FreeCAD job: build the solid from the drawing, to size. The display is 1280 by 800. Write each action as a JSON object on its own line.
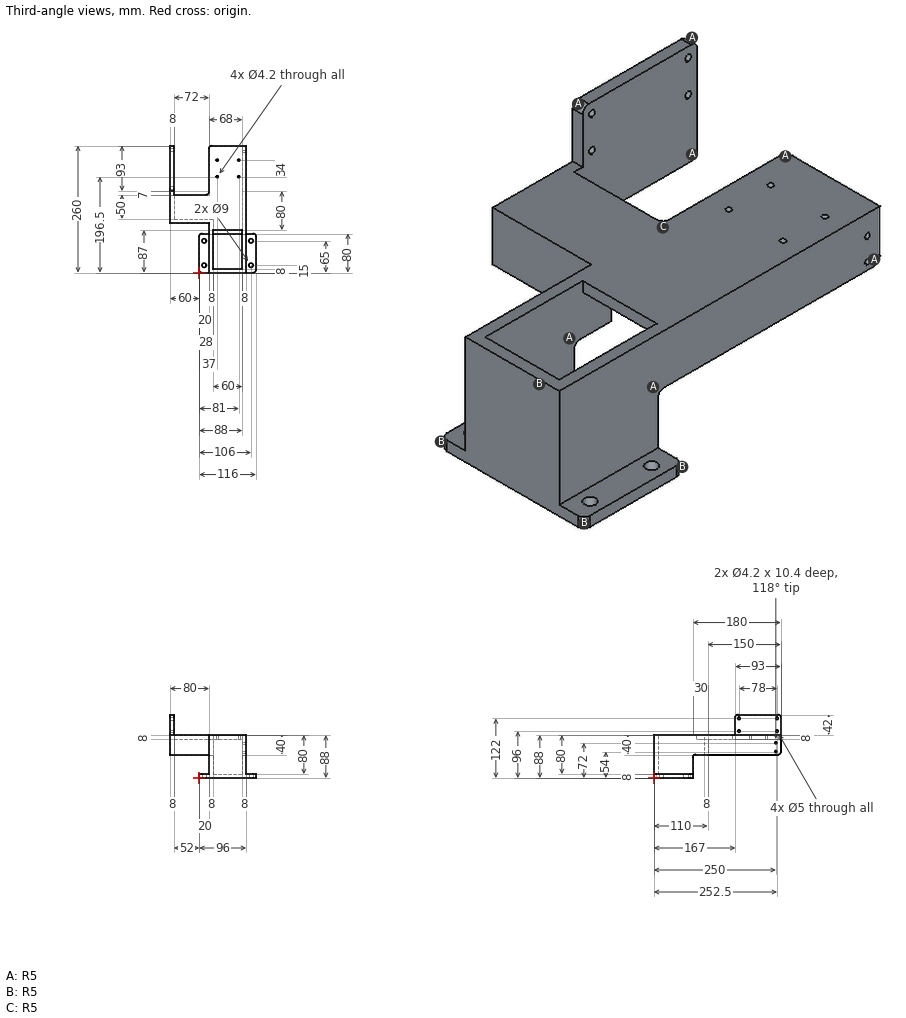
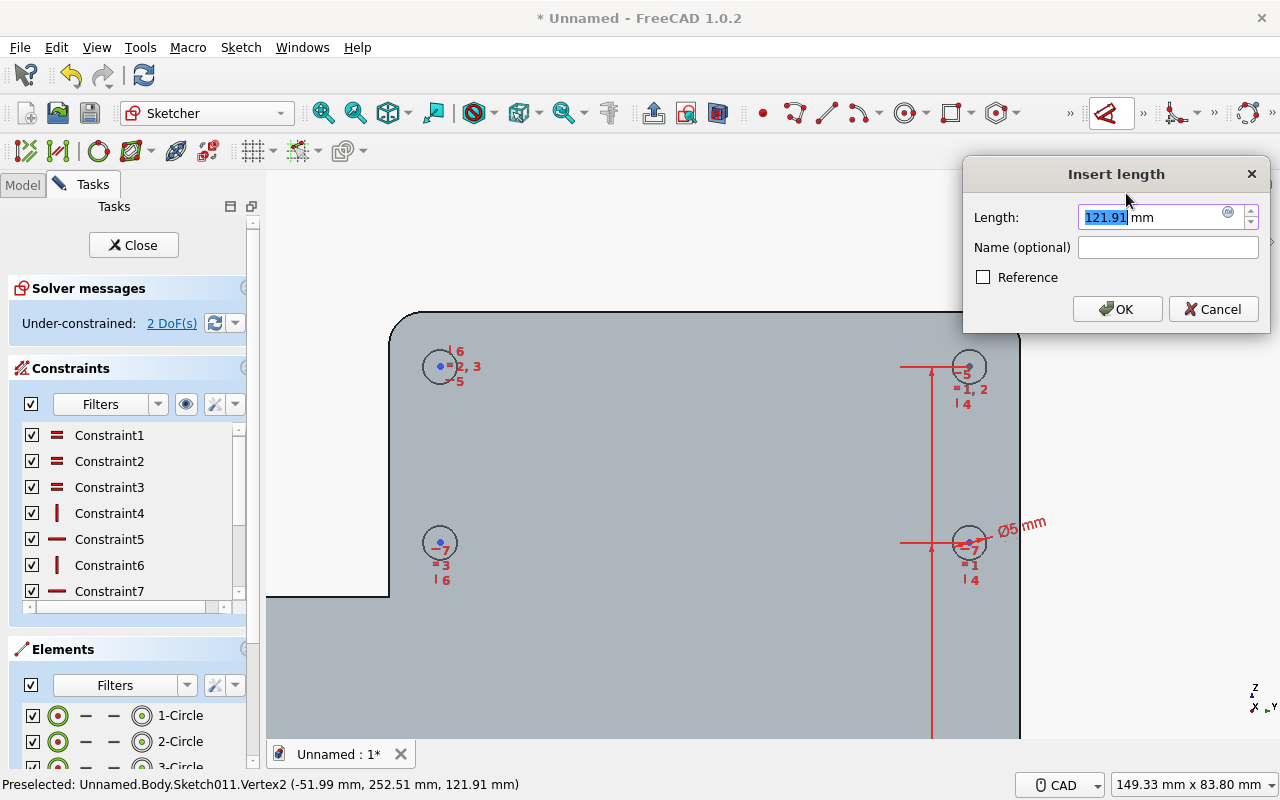
{"action": "type", "text": "122"}
{"action": "key", "text": "Return"}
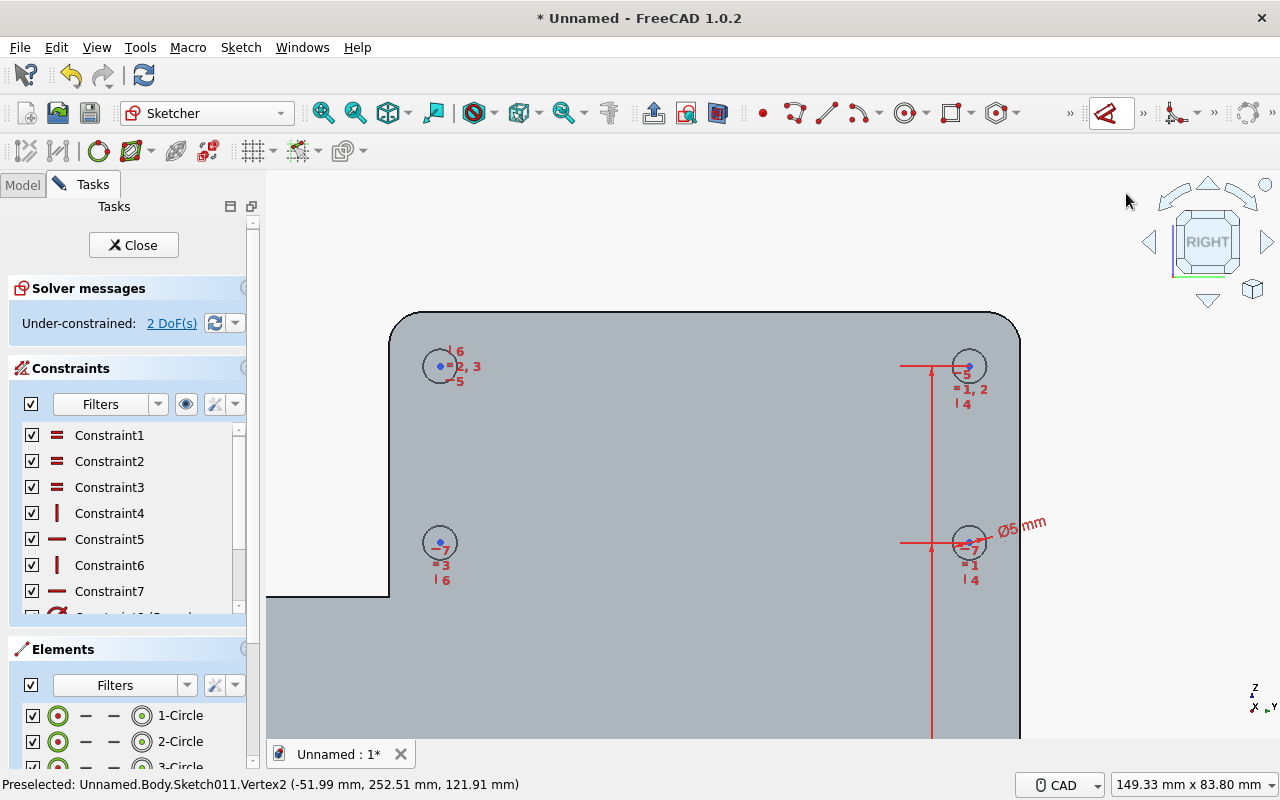
{"action": "left_click", "coordinate": [970, 366]}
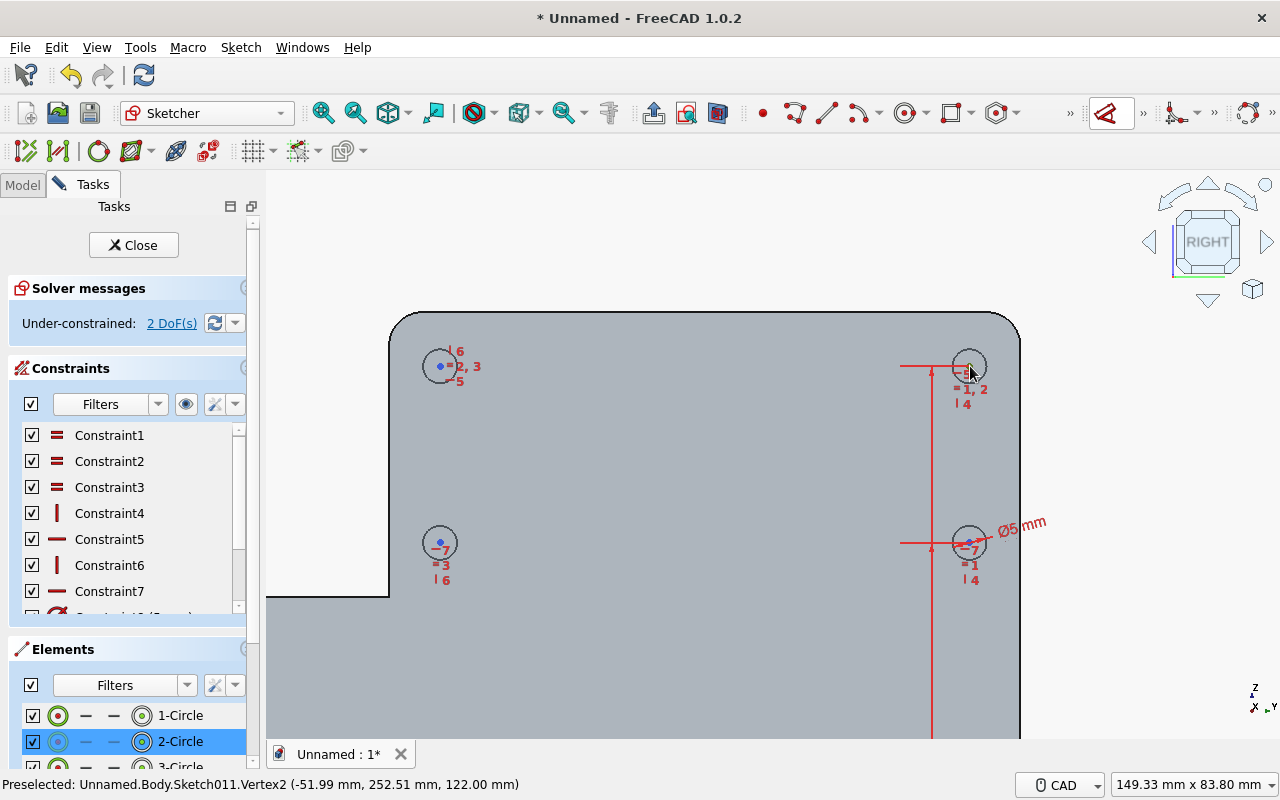
{"action": "left_click", "coordinate": [440, 366]}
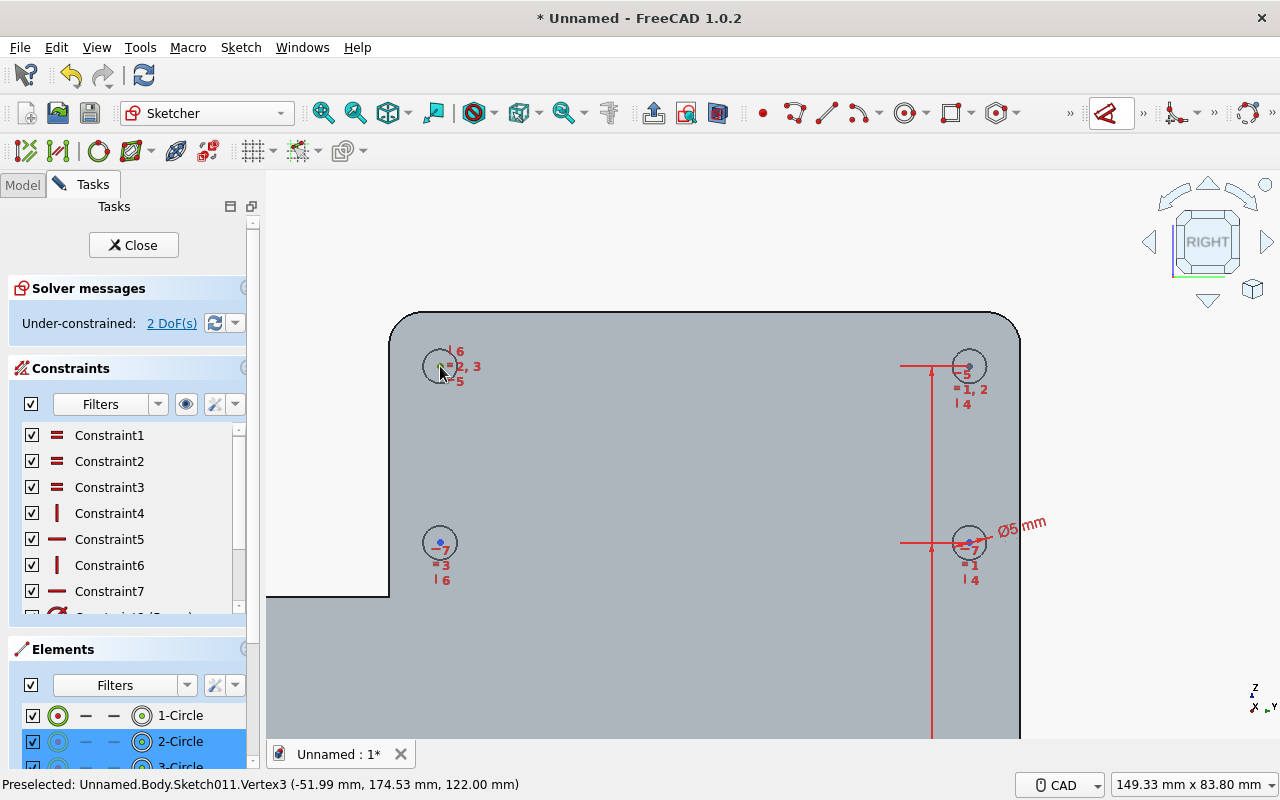
{"action": "left_click", "coordinate": [1128, 114]}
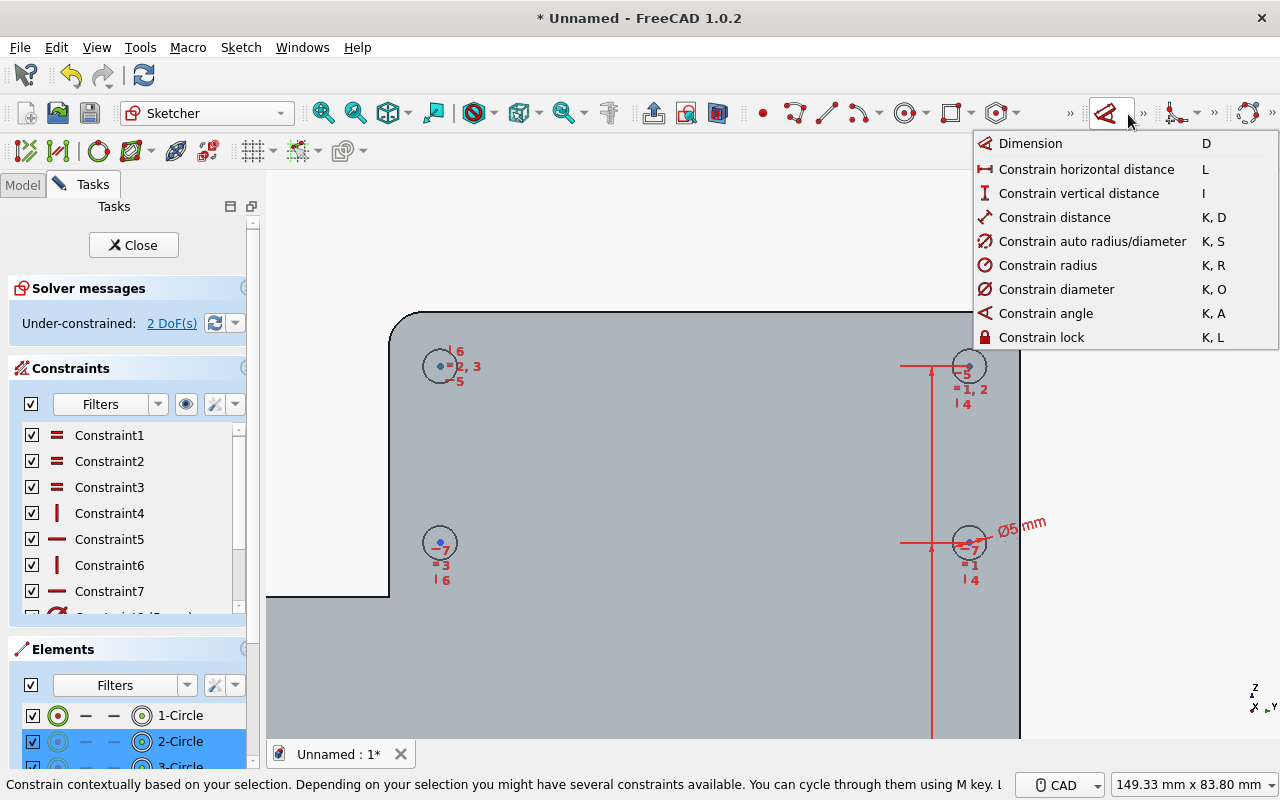
{"action": "left_click", "coordinate": [1126, 169]}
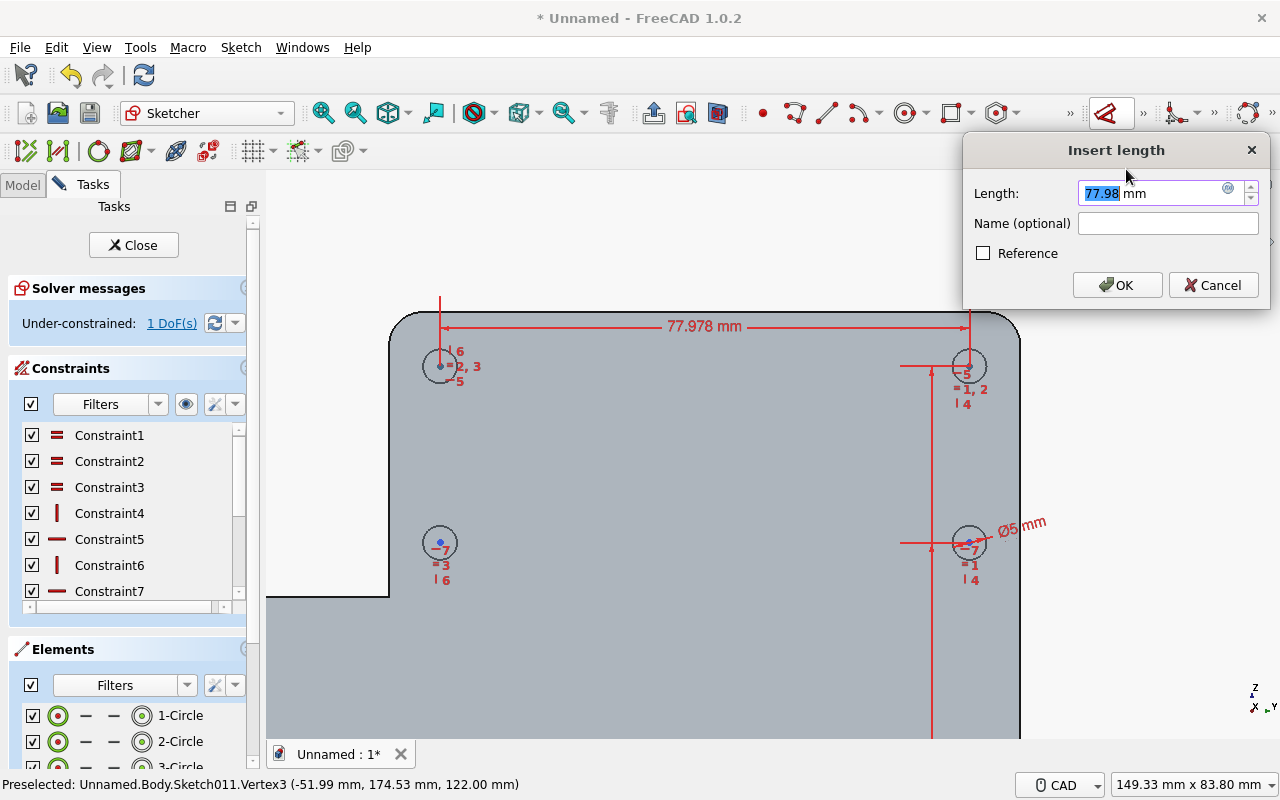
{"action": "type", "text": "78"}
{"action": "key", "text": "Return"}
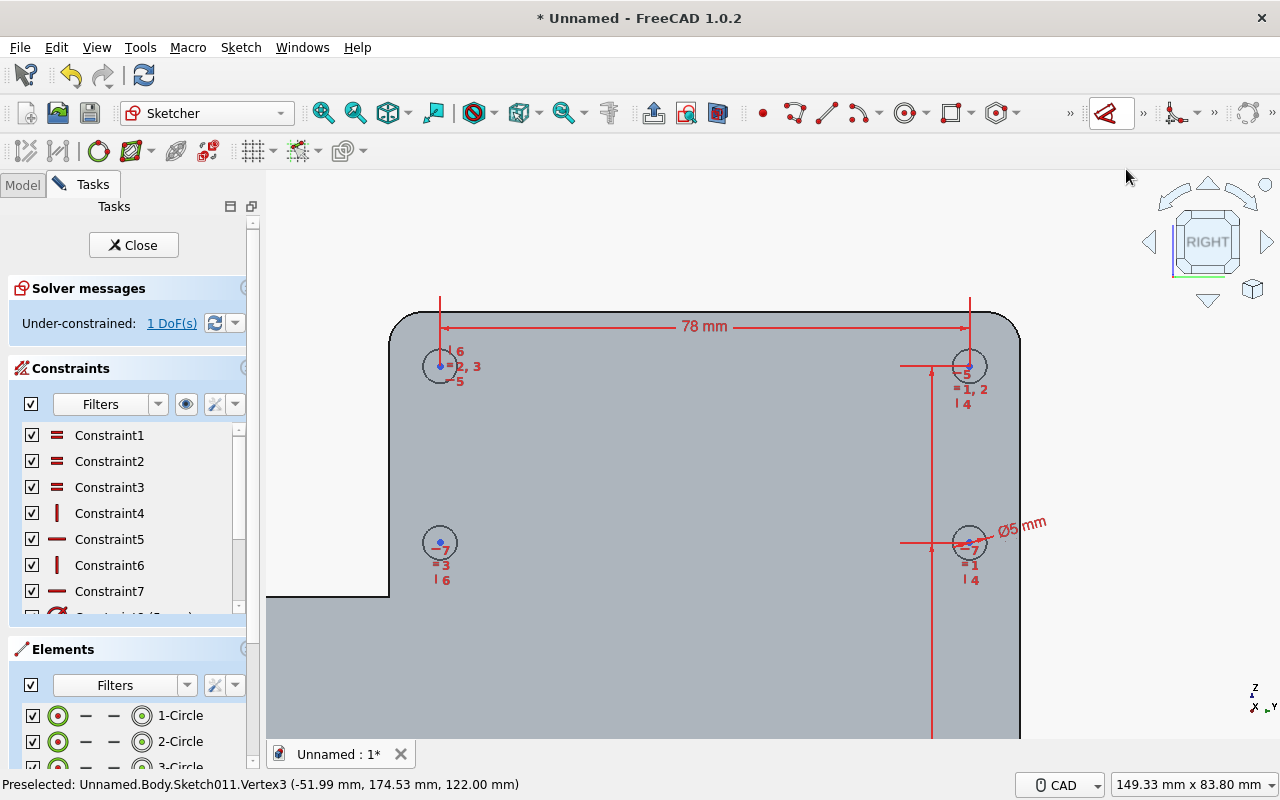
{"action": "left_click", "coordinate": [970, 543]}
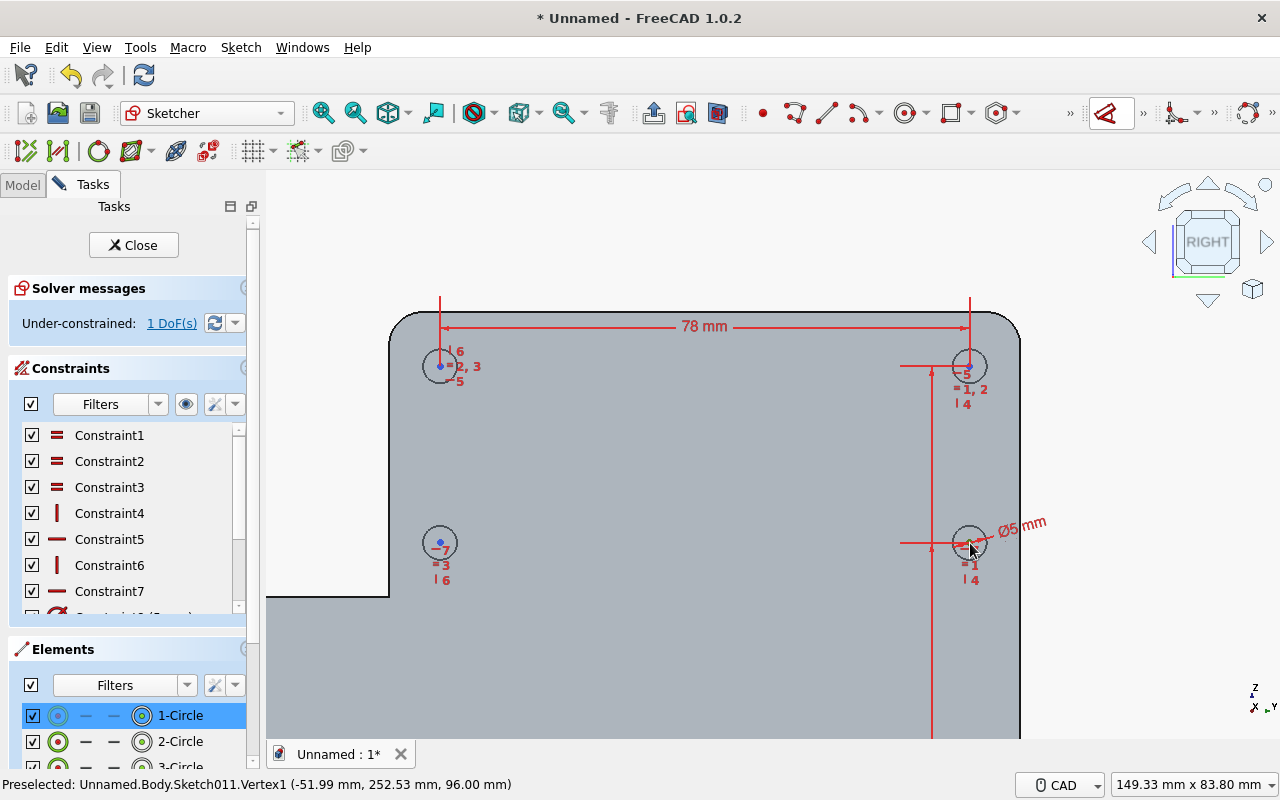
{"action": "key", "text": "l"}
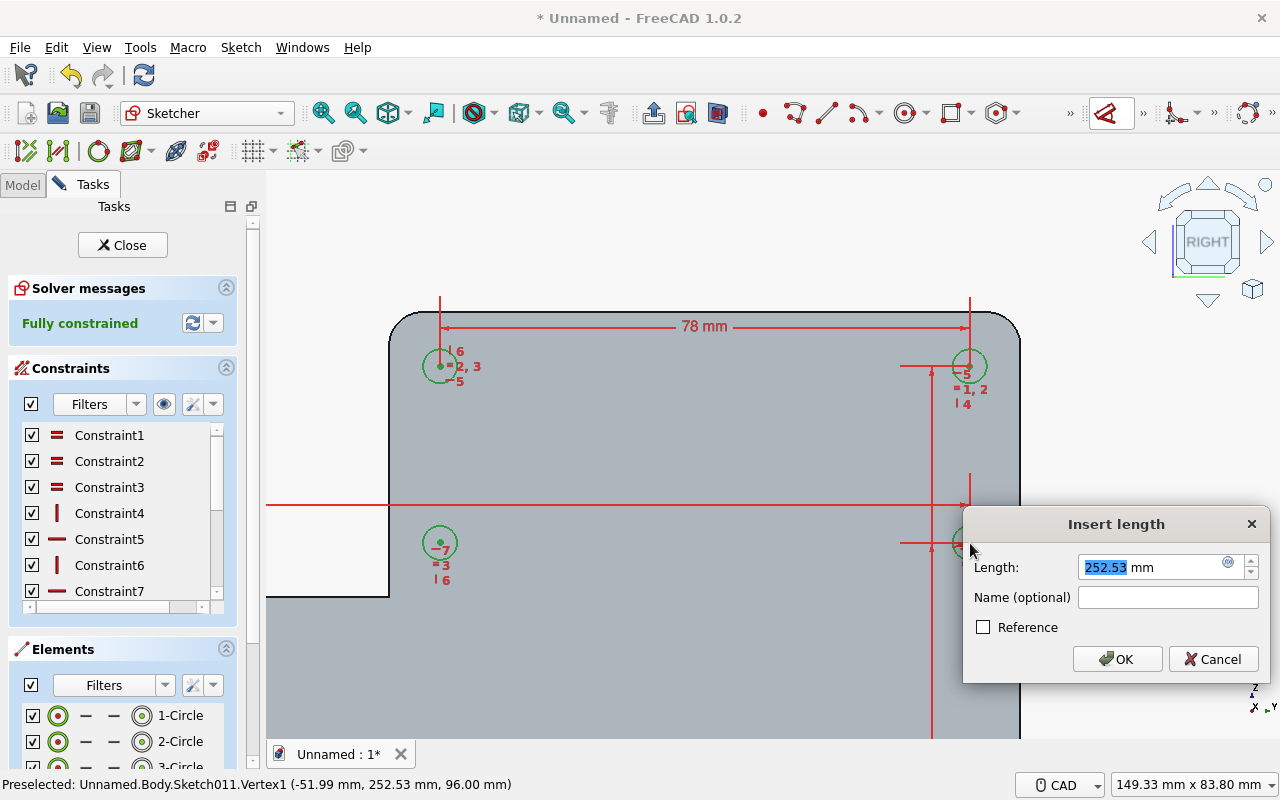
{"action": "type", "text": "252.5"}
{"action": "key", "text": "Return"}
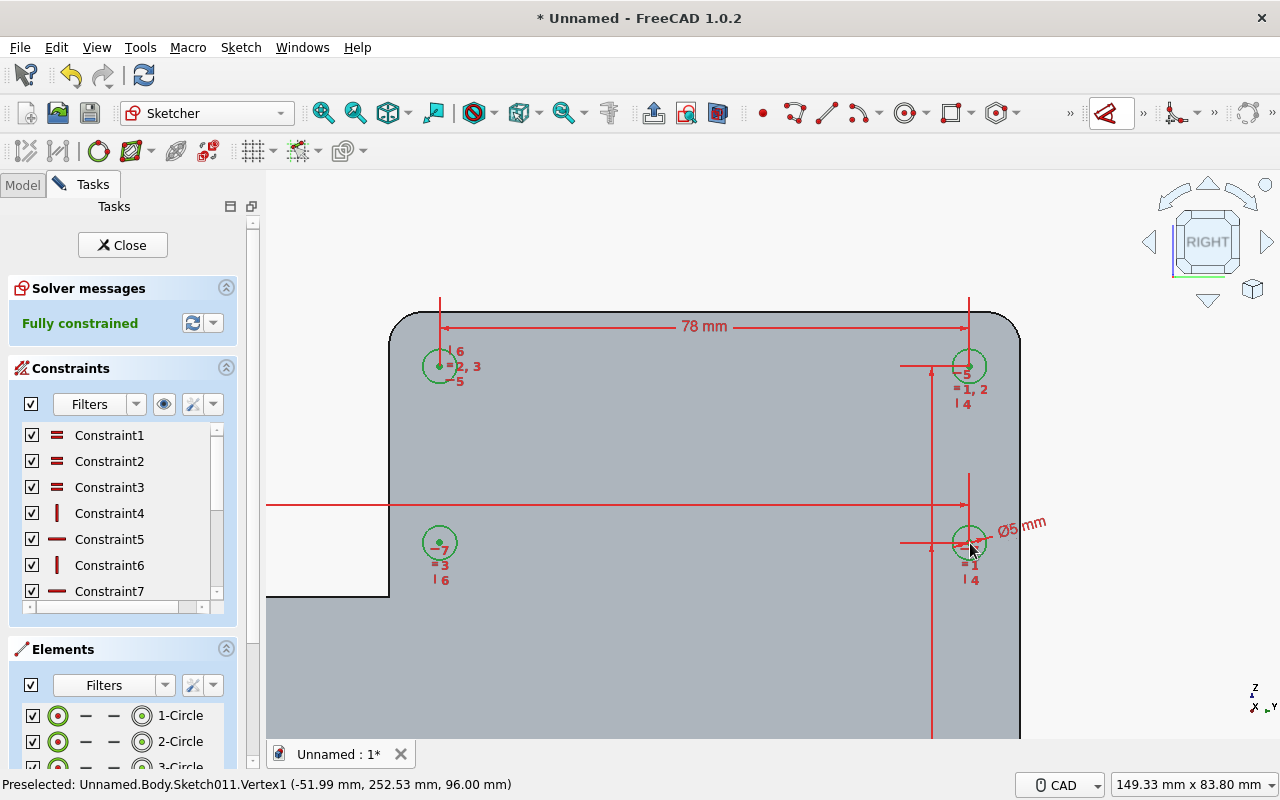
{"action": "left_click", "coordinate": [123, 245]}